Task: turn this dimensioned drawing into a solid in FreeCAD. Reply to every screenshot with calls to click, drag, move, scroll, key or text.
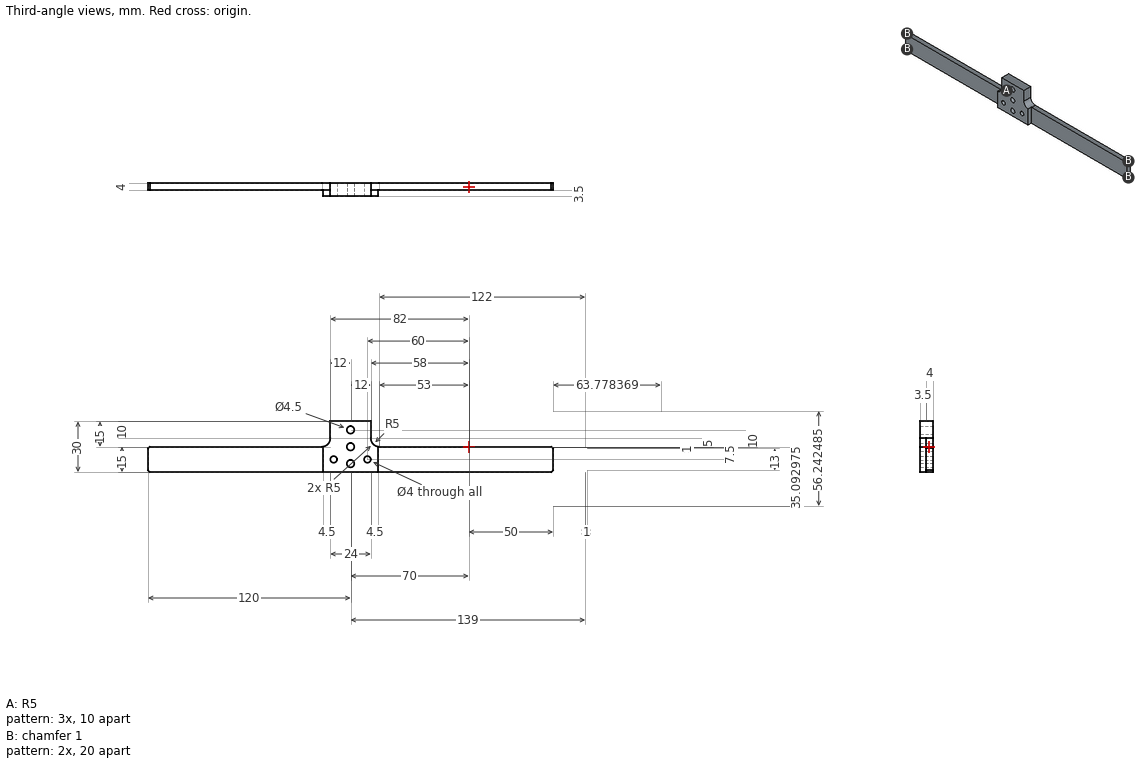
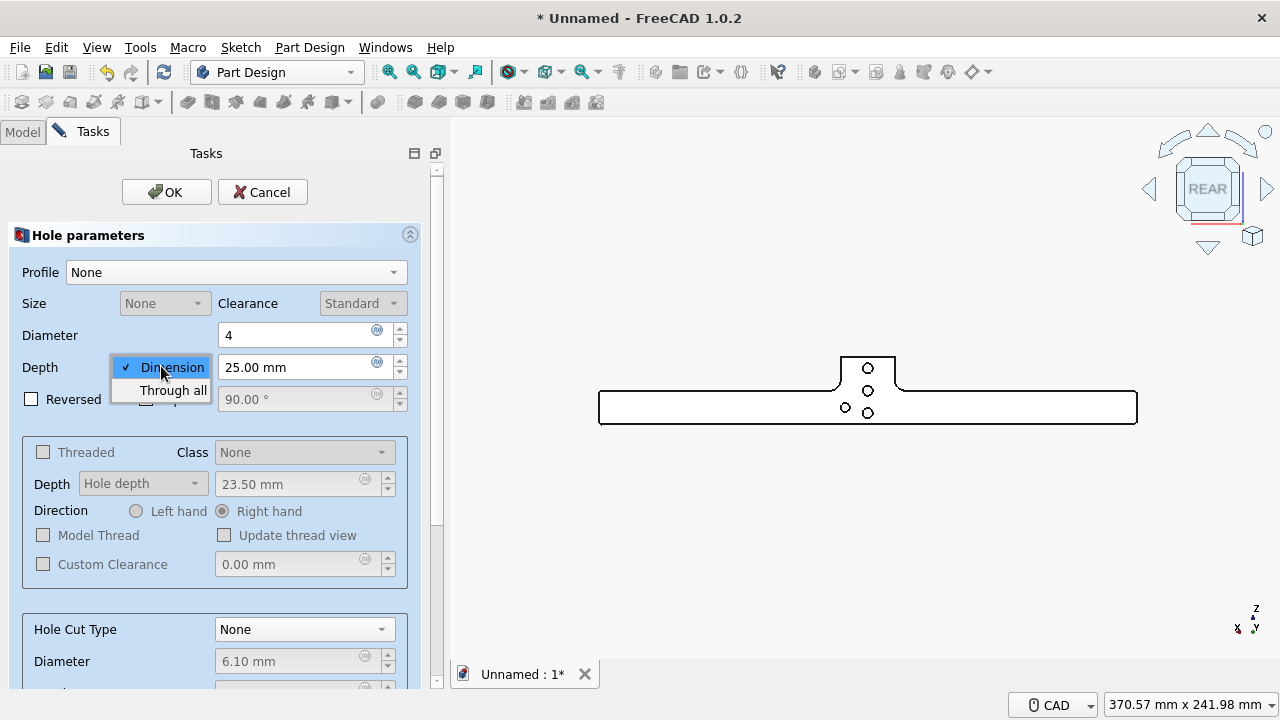
click(160, 390)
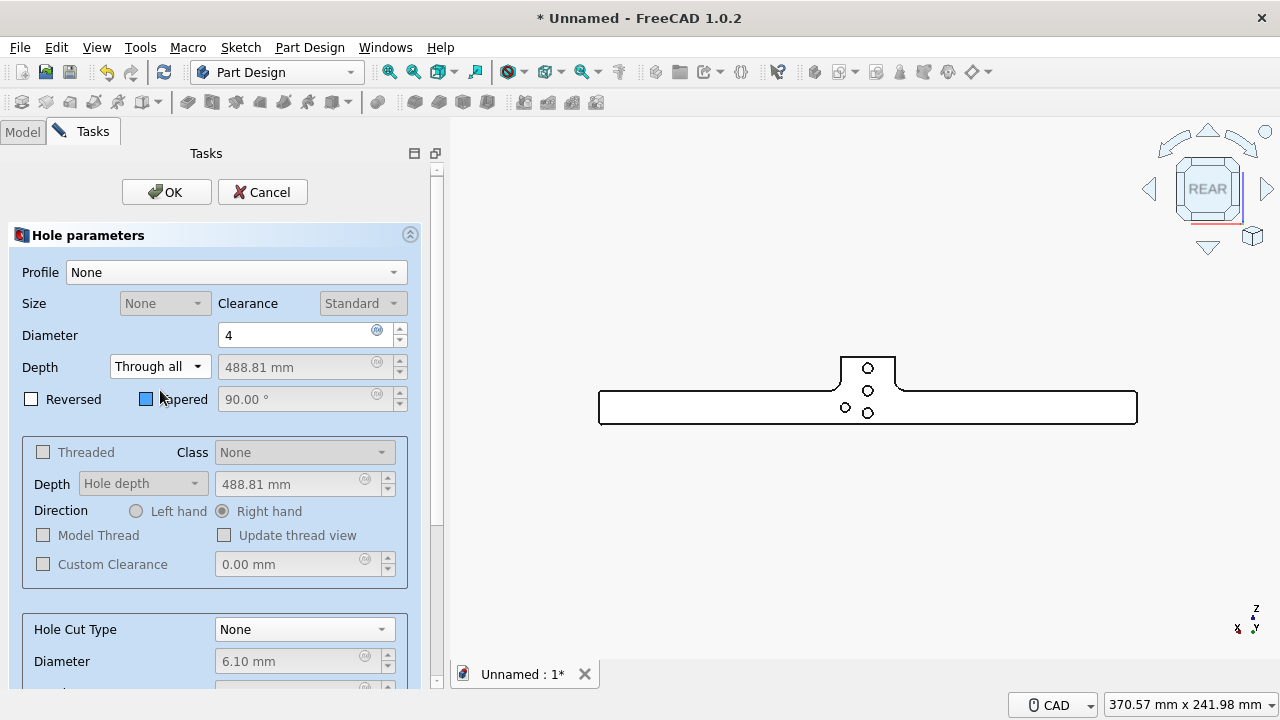
click(167, 192)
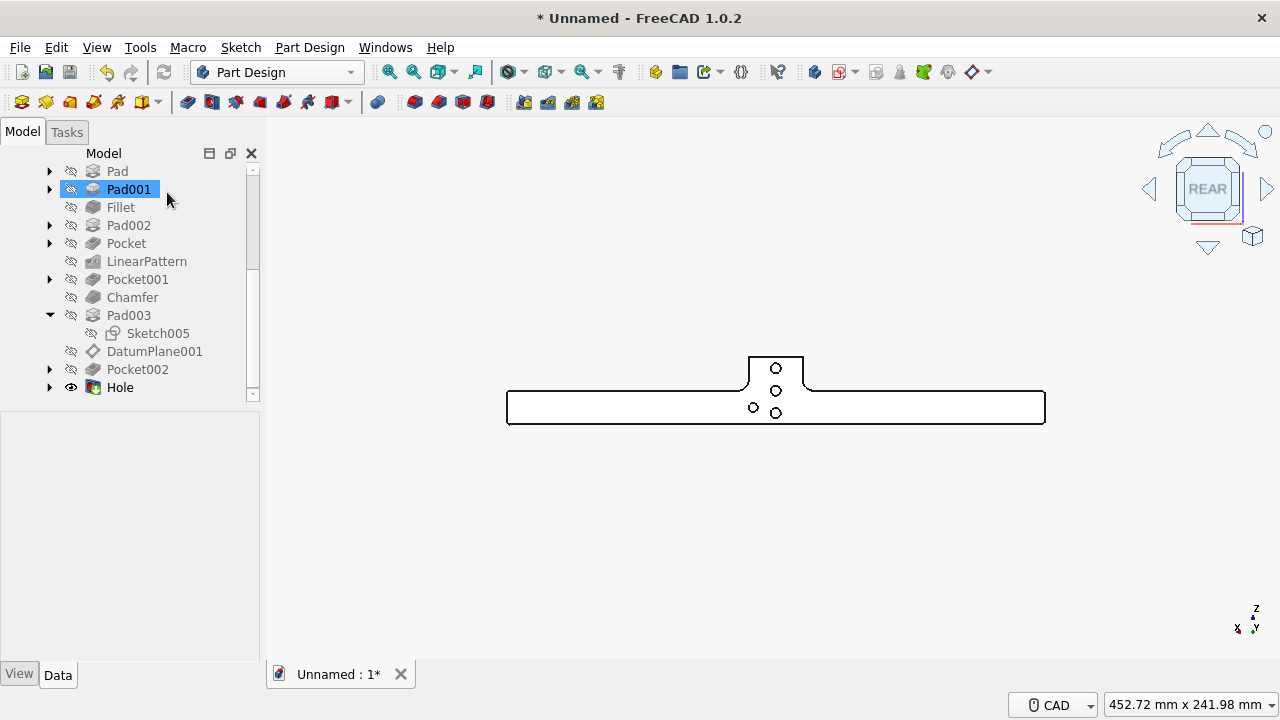
click(116, 387)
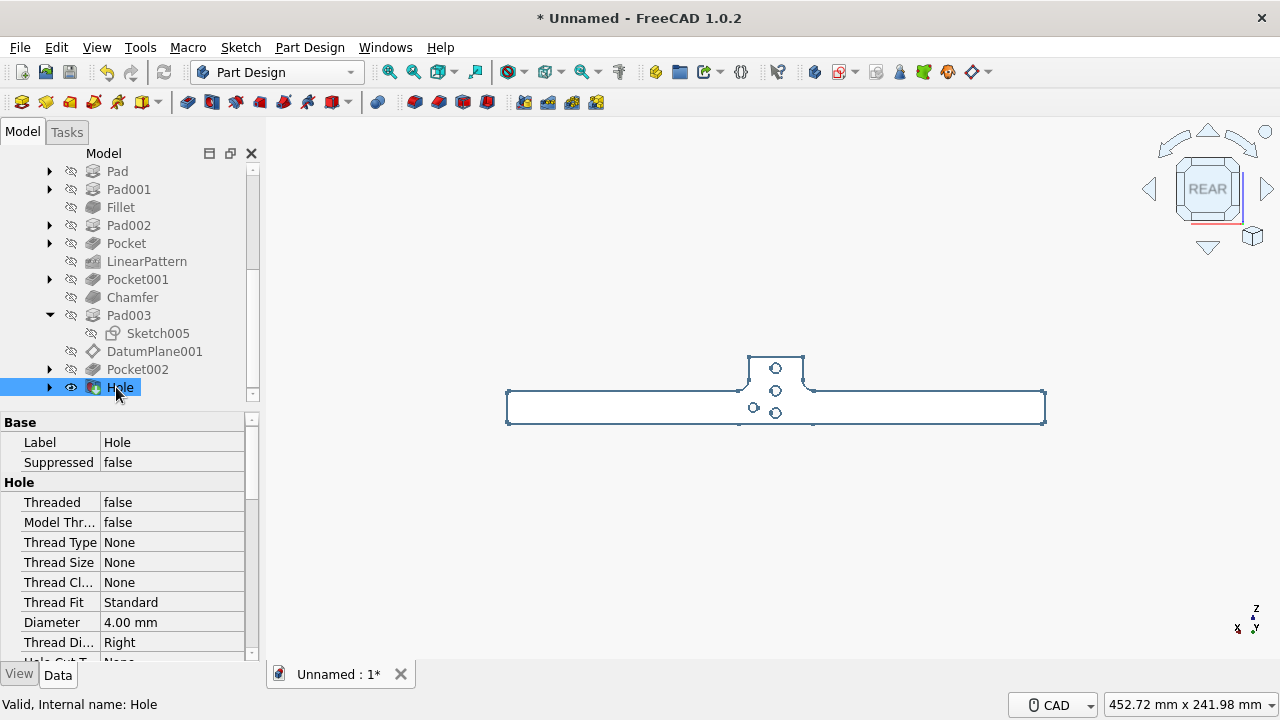
click(548, 102)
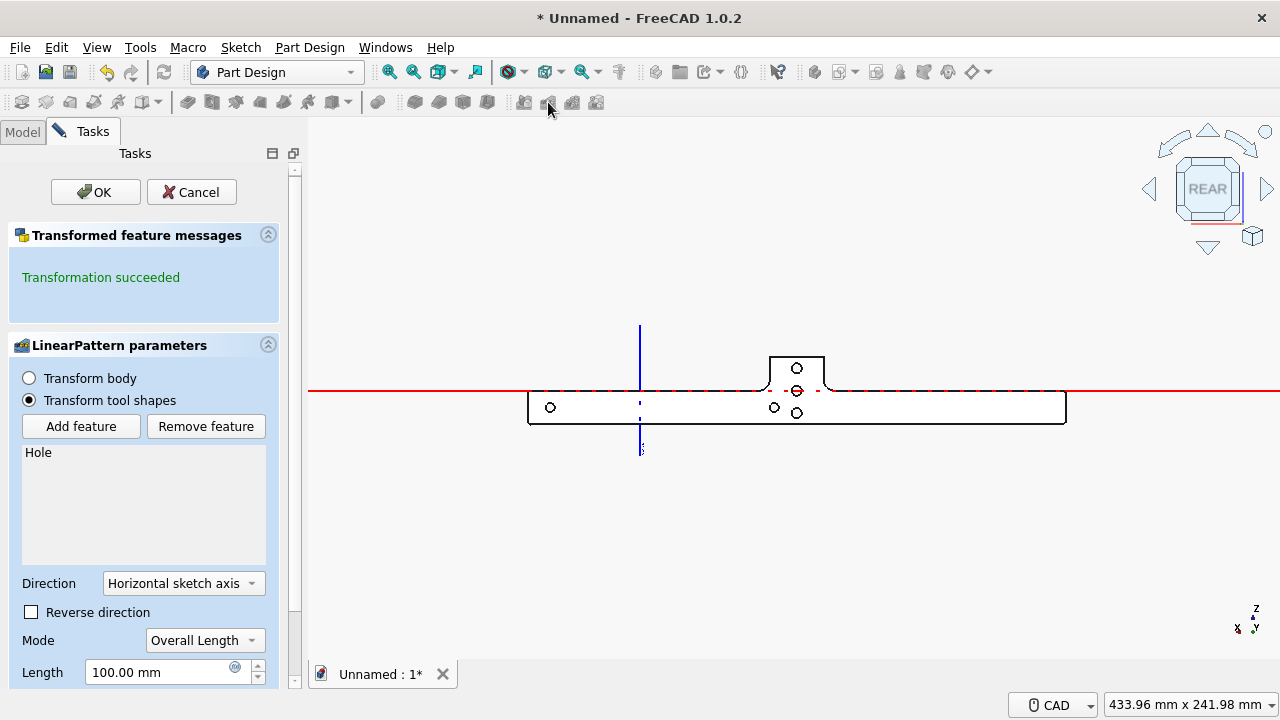
click(184, 584)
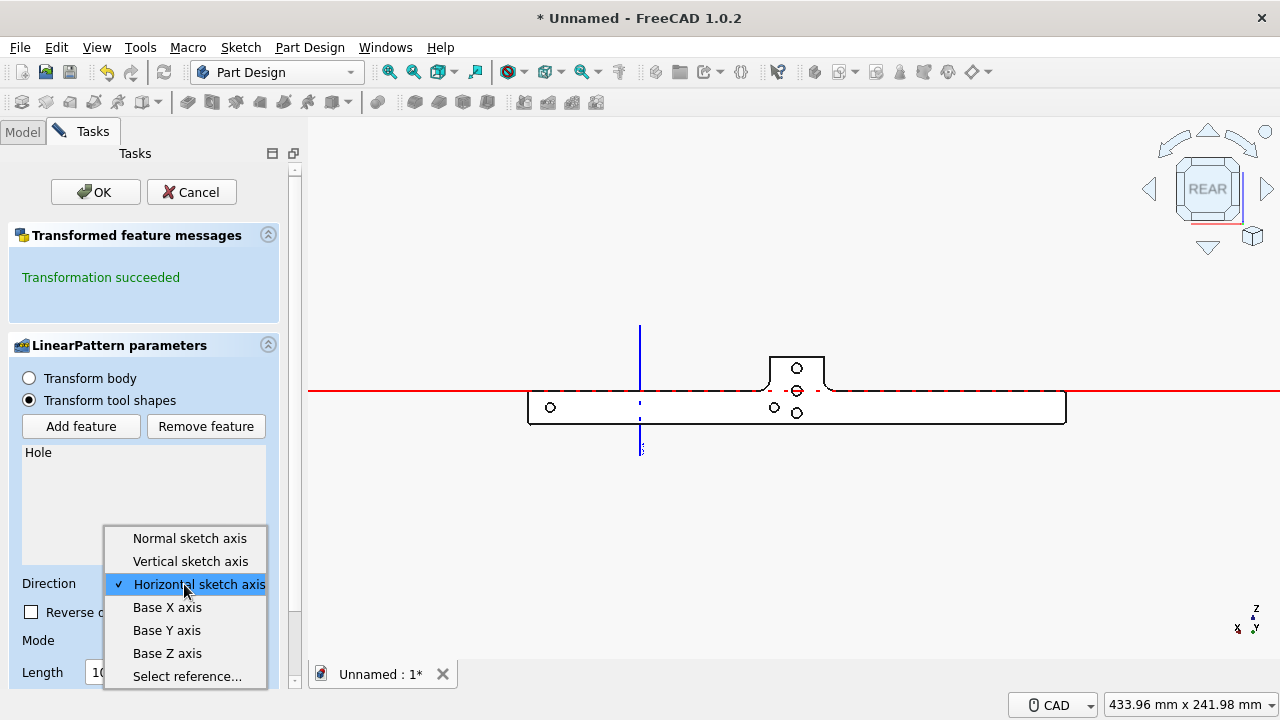
click(184, 608)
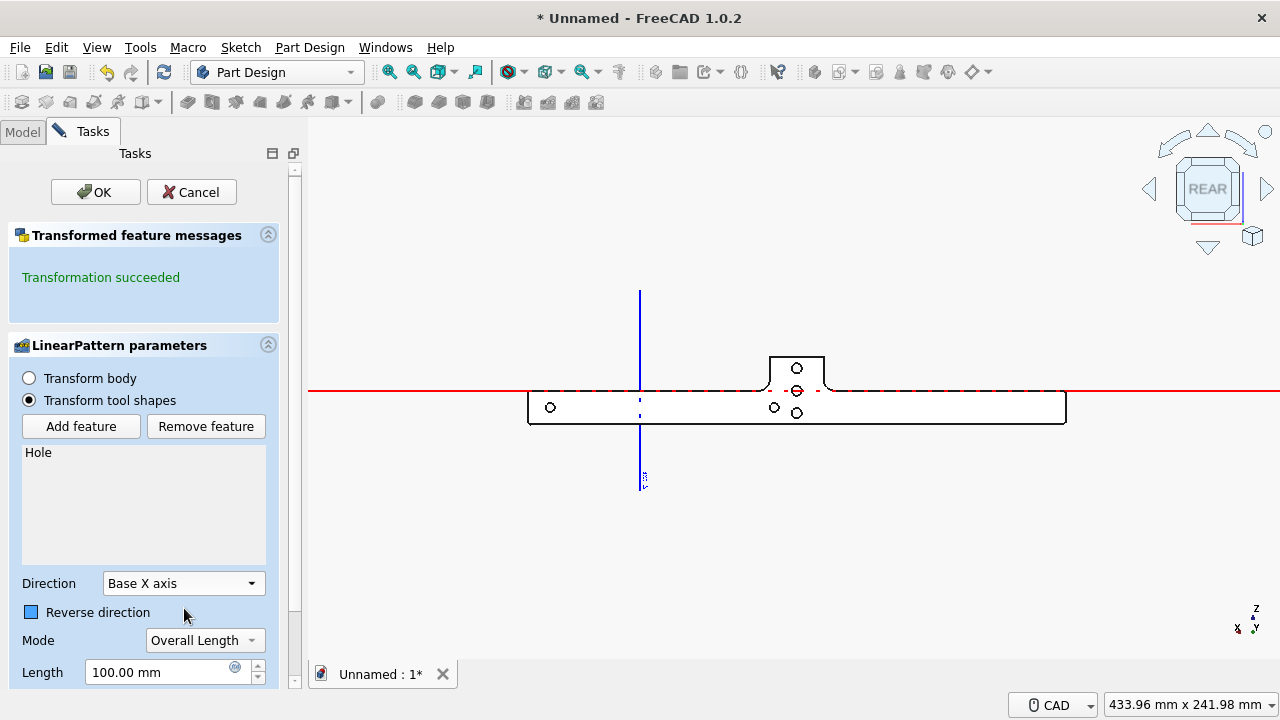
click(206, 640)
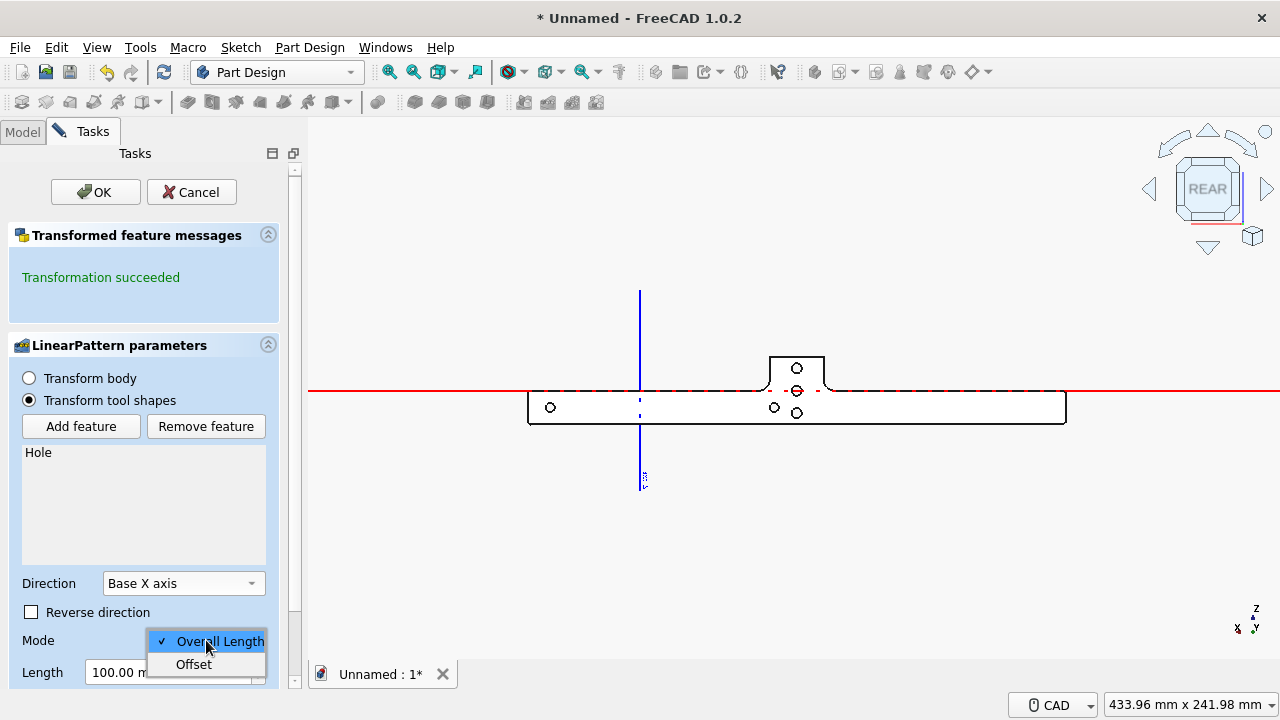
click(206, 664)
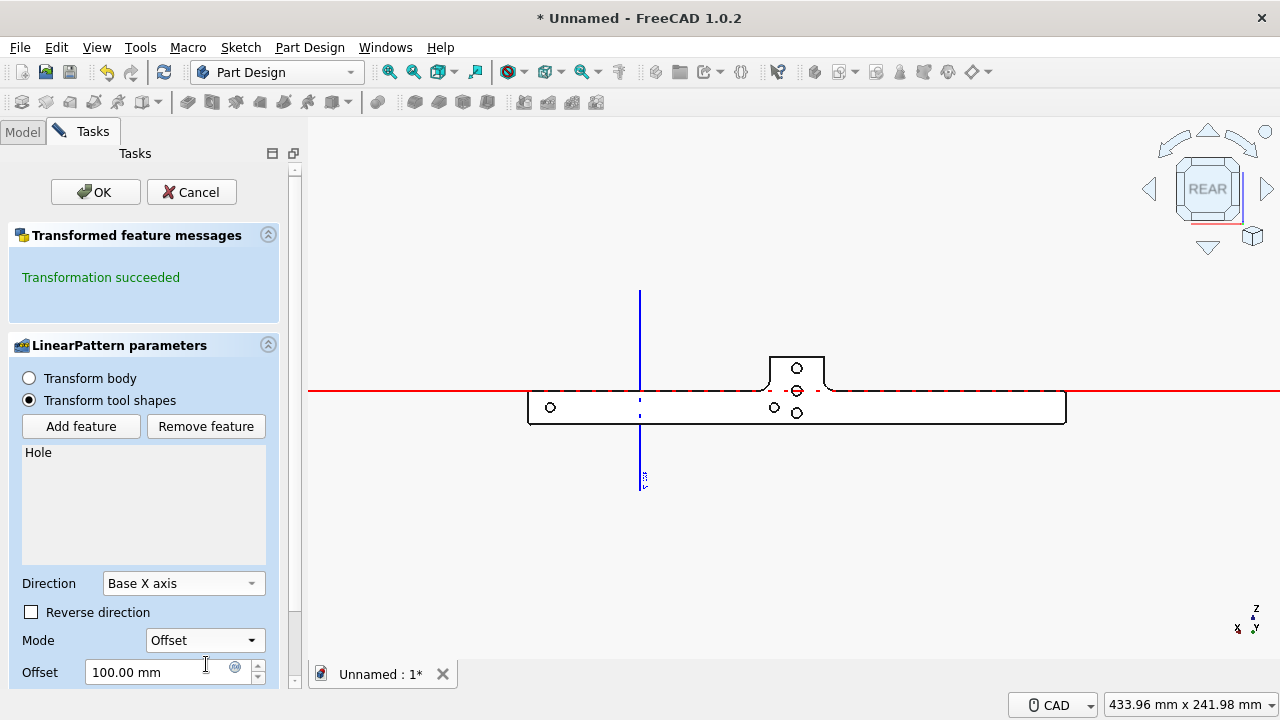
triple_click(168, 672)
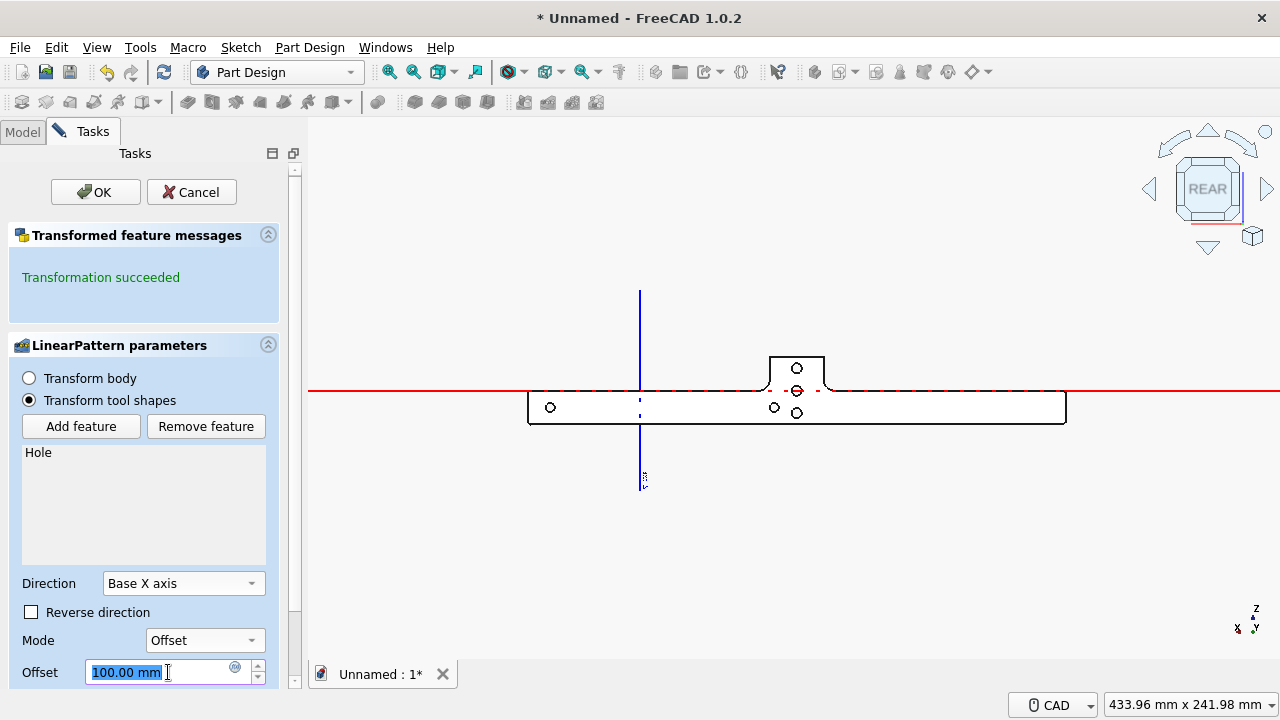
text(20)
key(Tab)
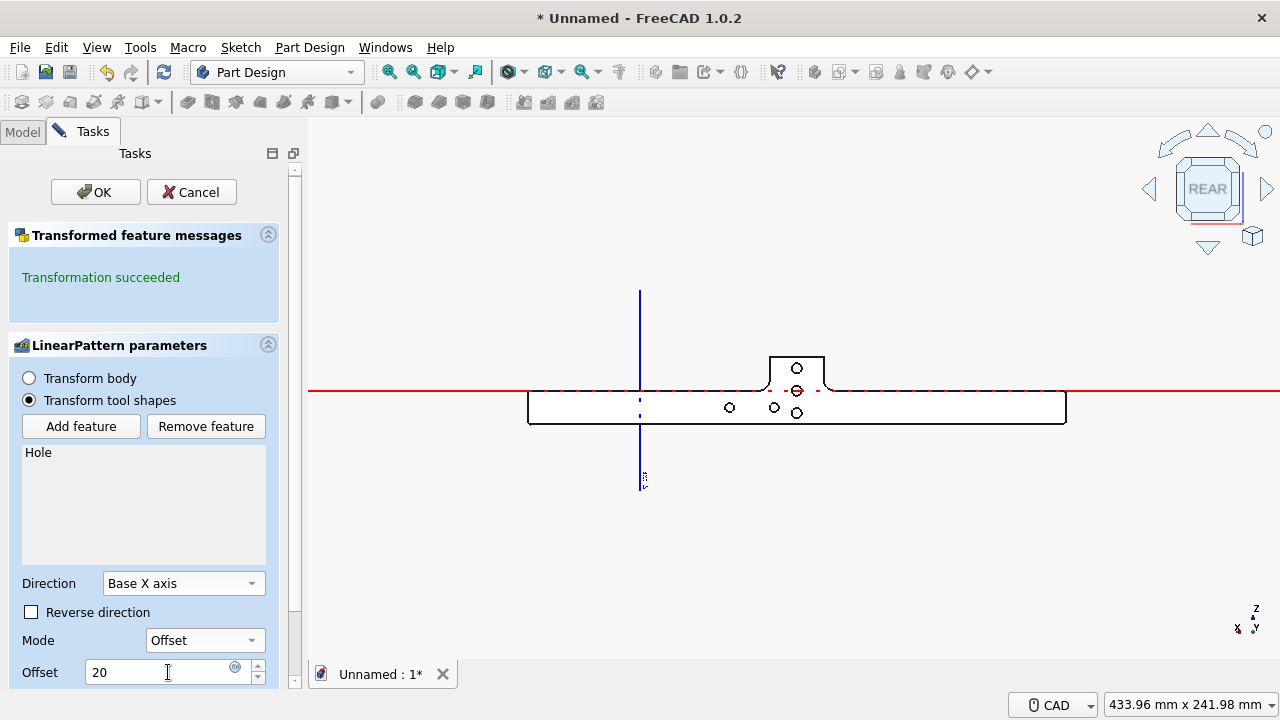
scroll(295, 426, down, 2)